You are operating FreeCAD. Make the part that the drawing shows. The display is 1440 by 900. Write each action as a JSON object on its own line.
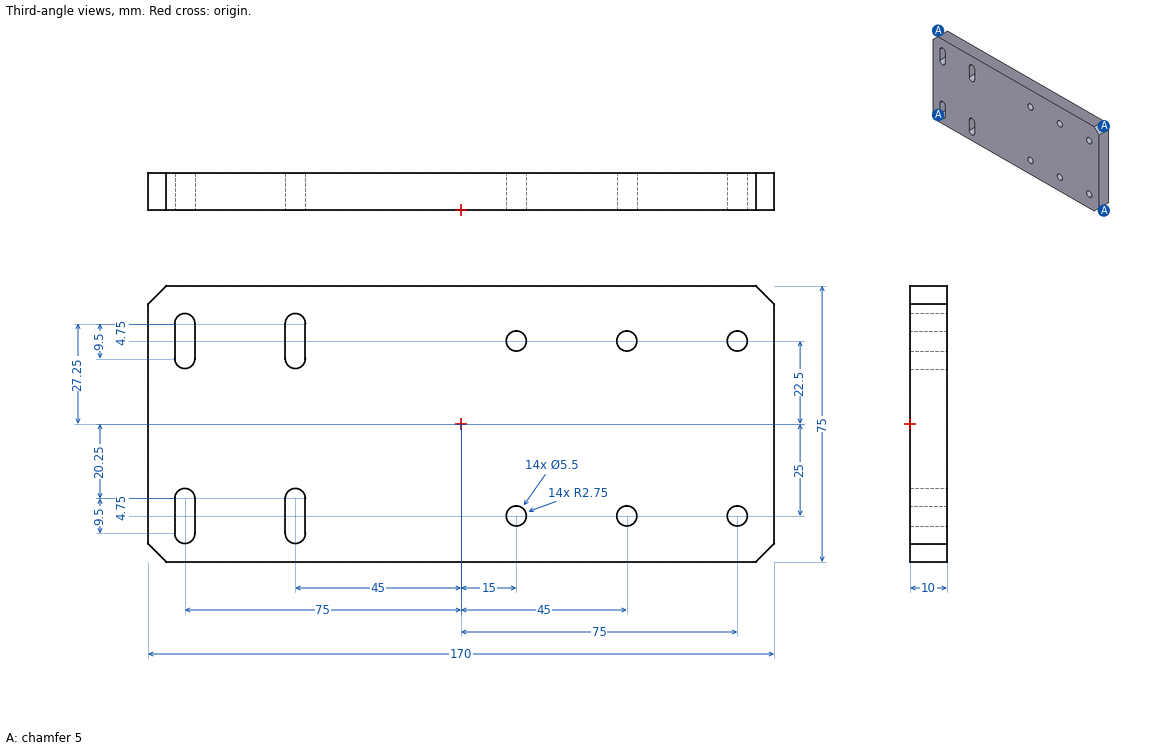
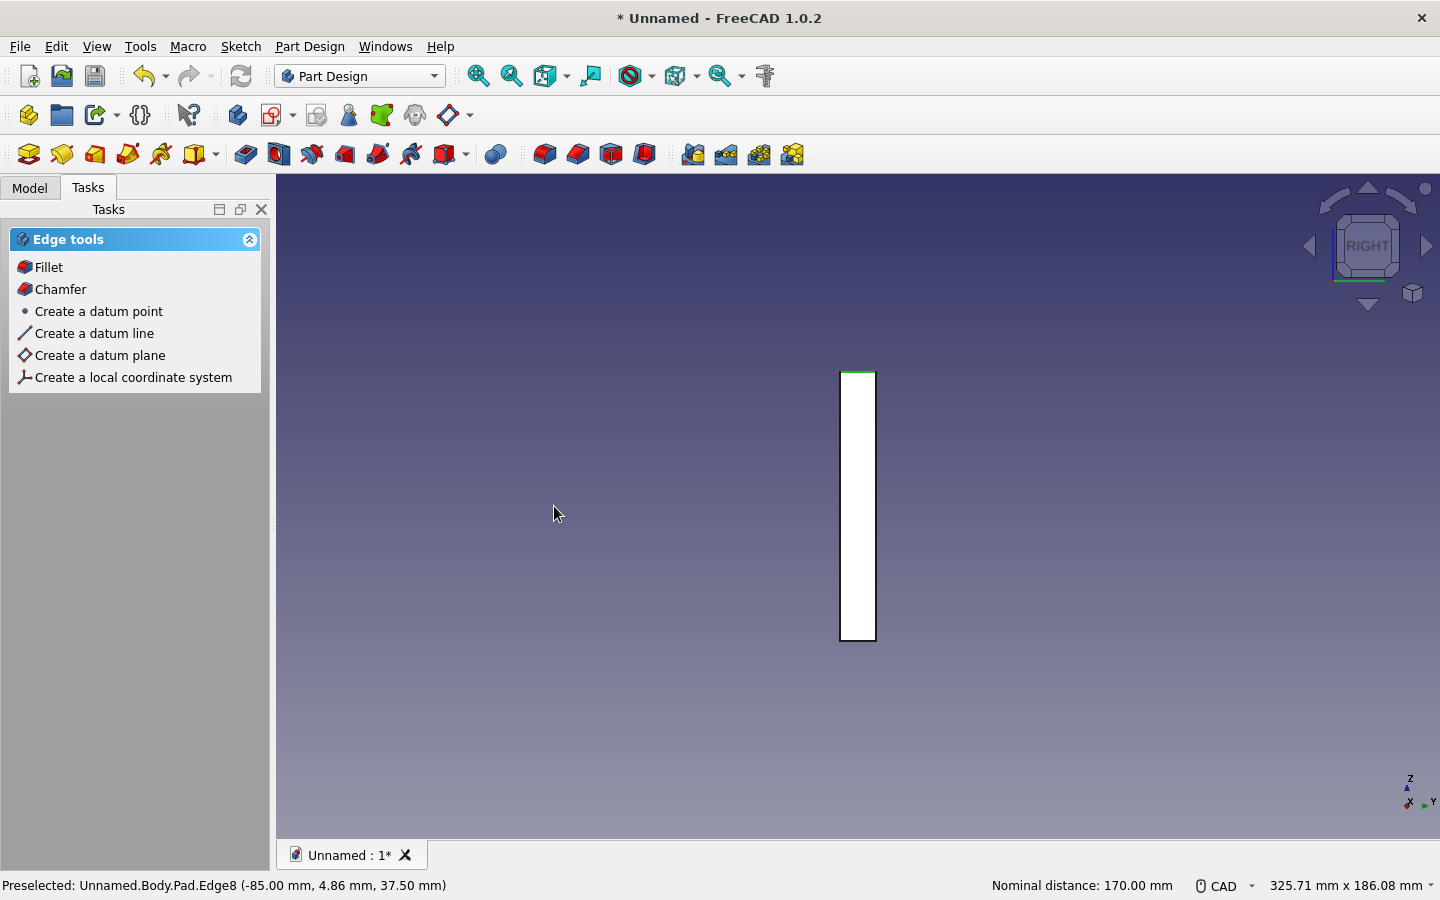
{"action": "key", "text": "v f"}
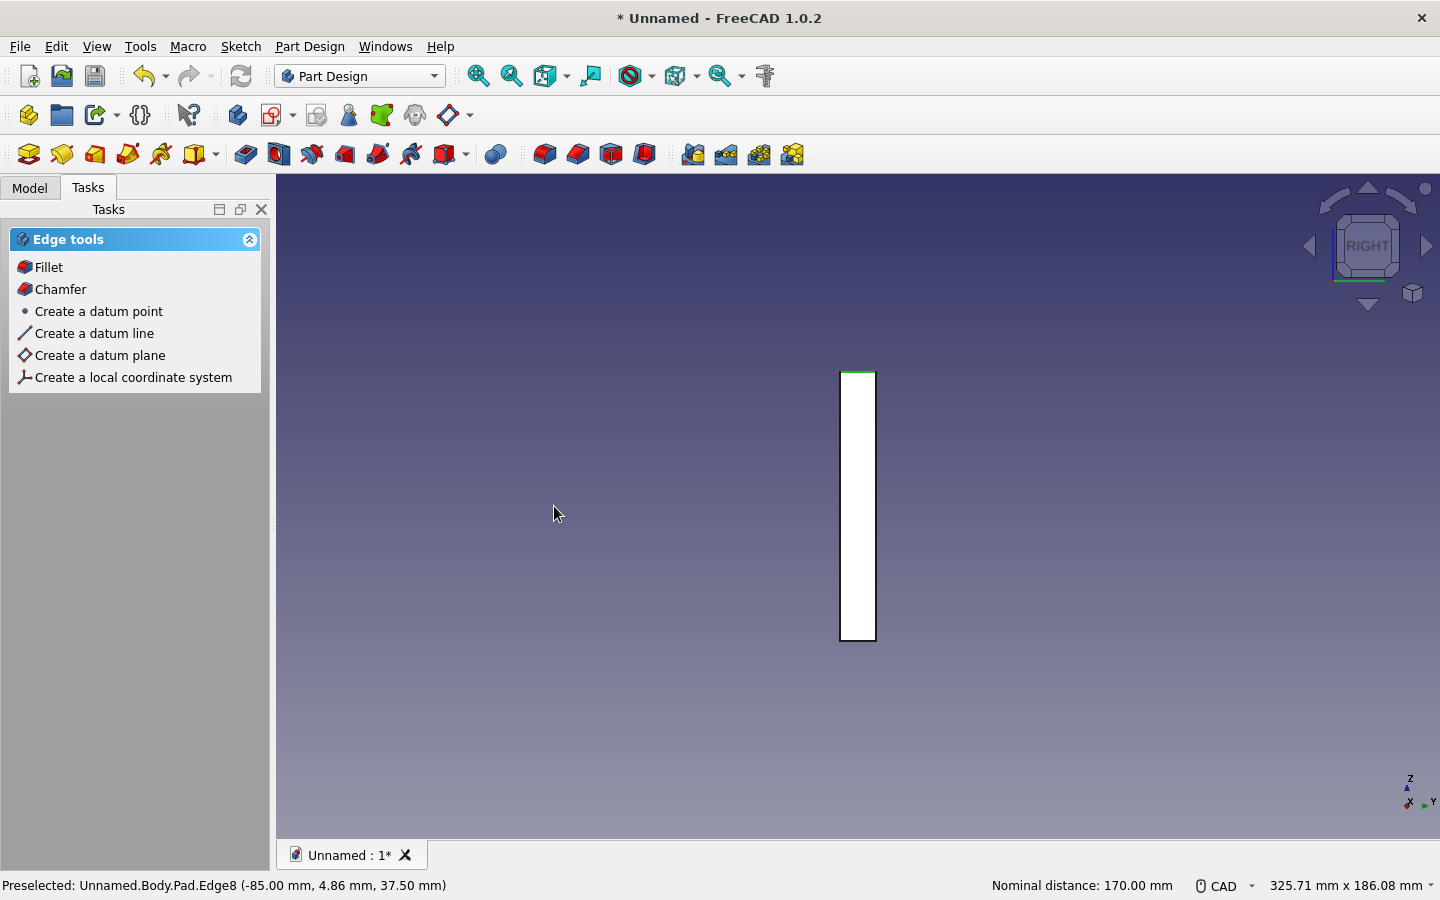
{"action": "left_click", "coordinate": [858, 640], "text": "ctrl"}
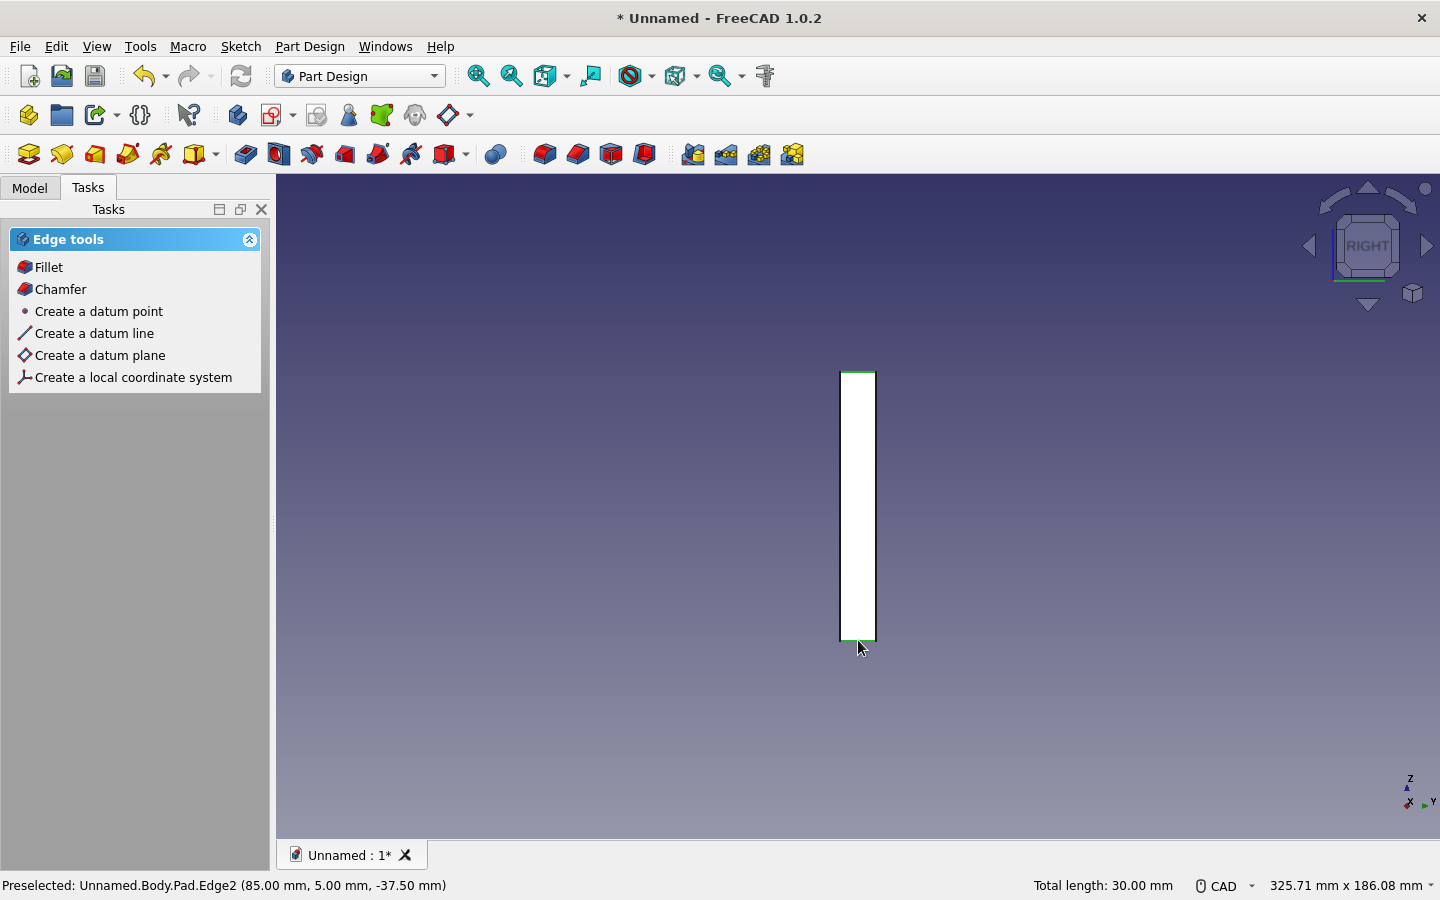
{"action": "key", "text": "5"}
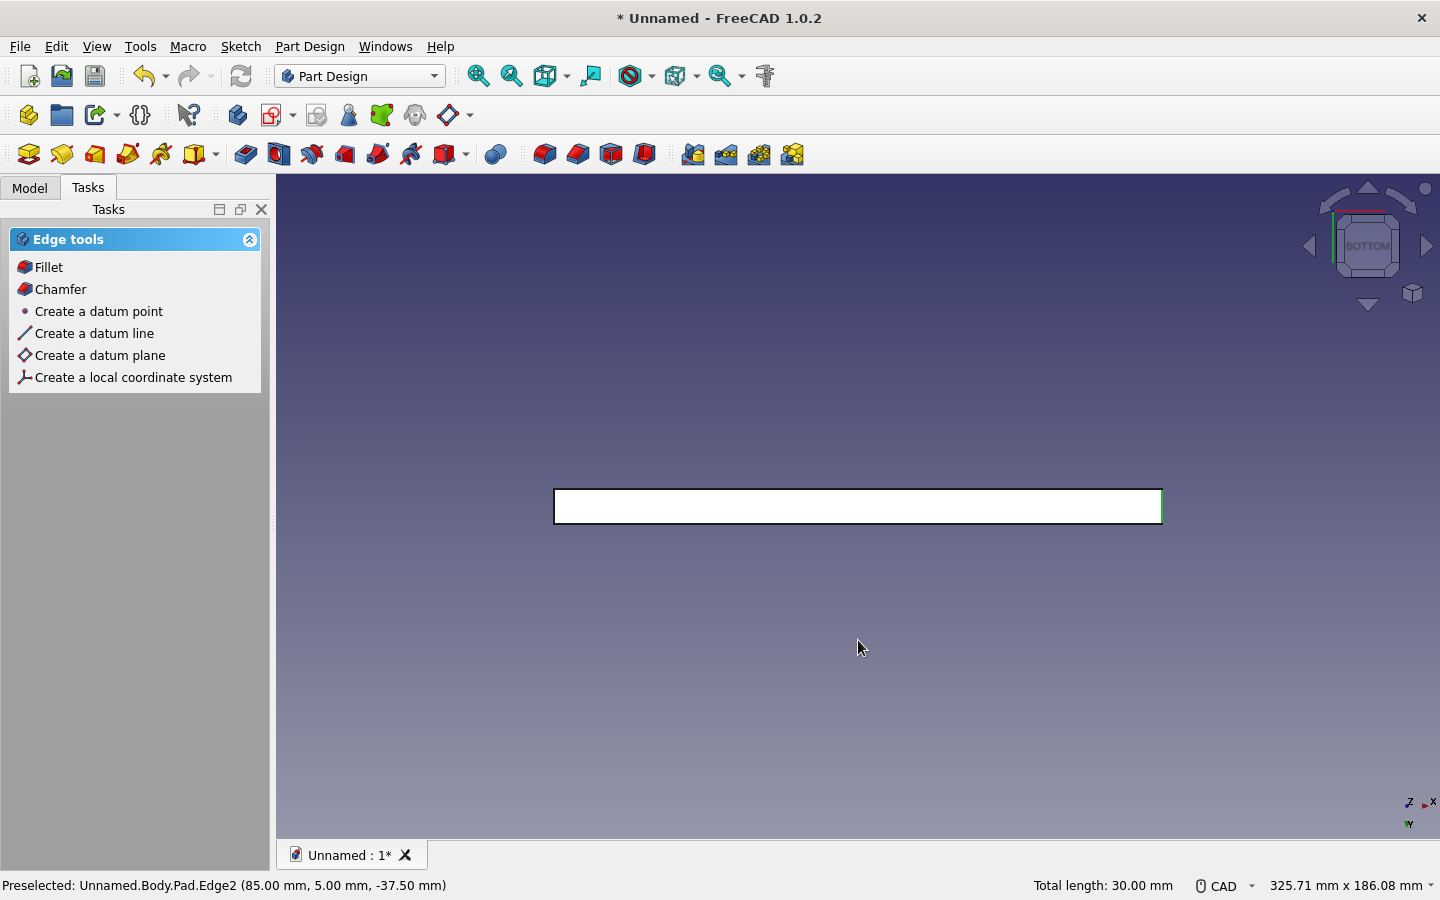
{"action": "left_click", "coordinate": [554, 505], "text": "ctrl"}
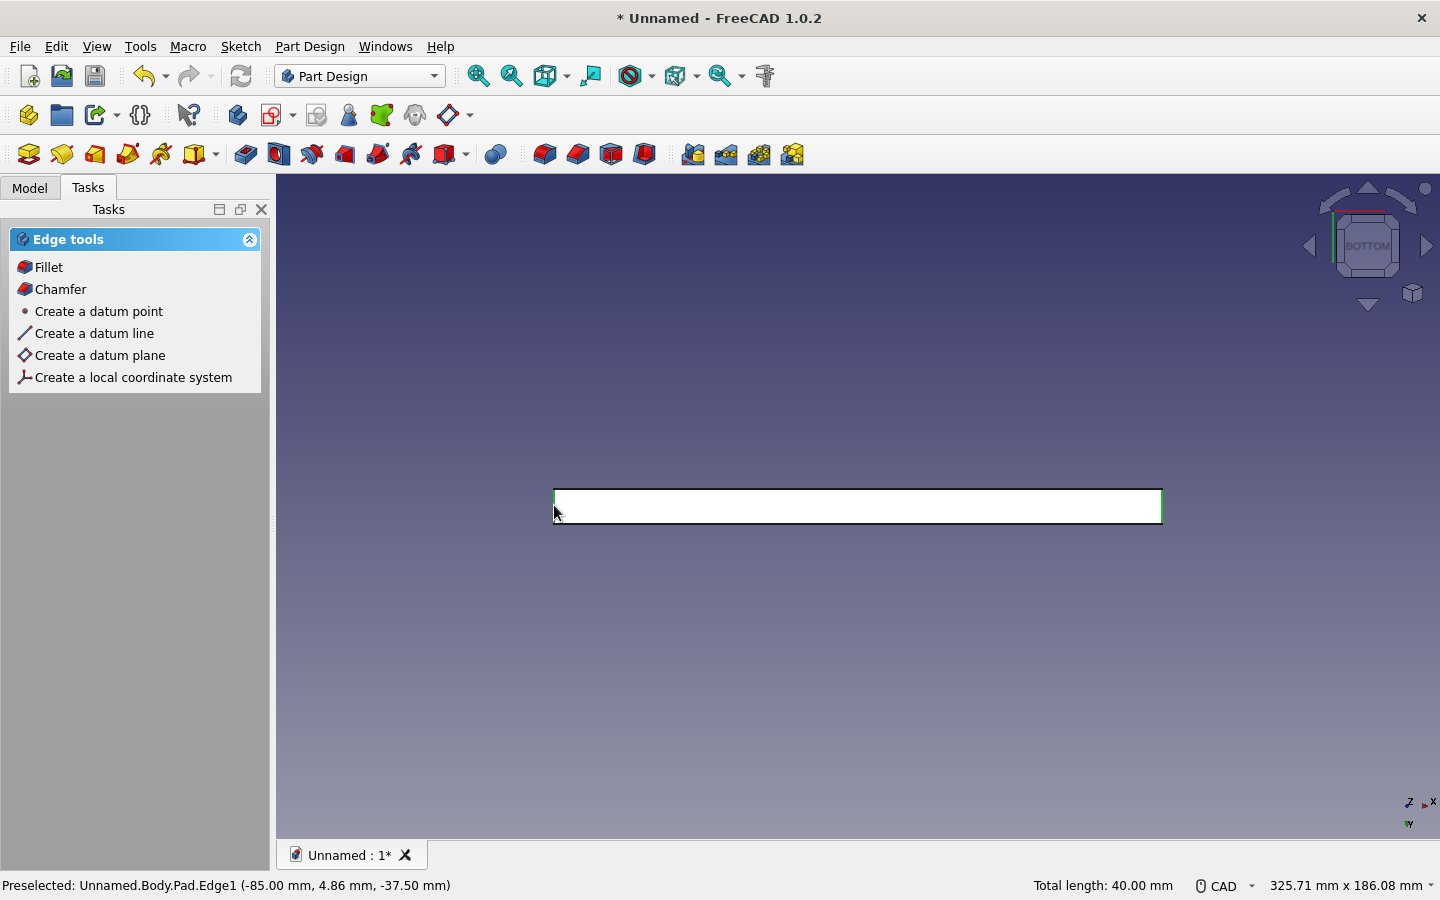
{"action": "left_click", "coordinate": [578, 154]}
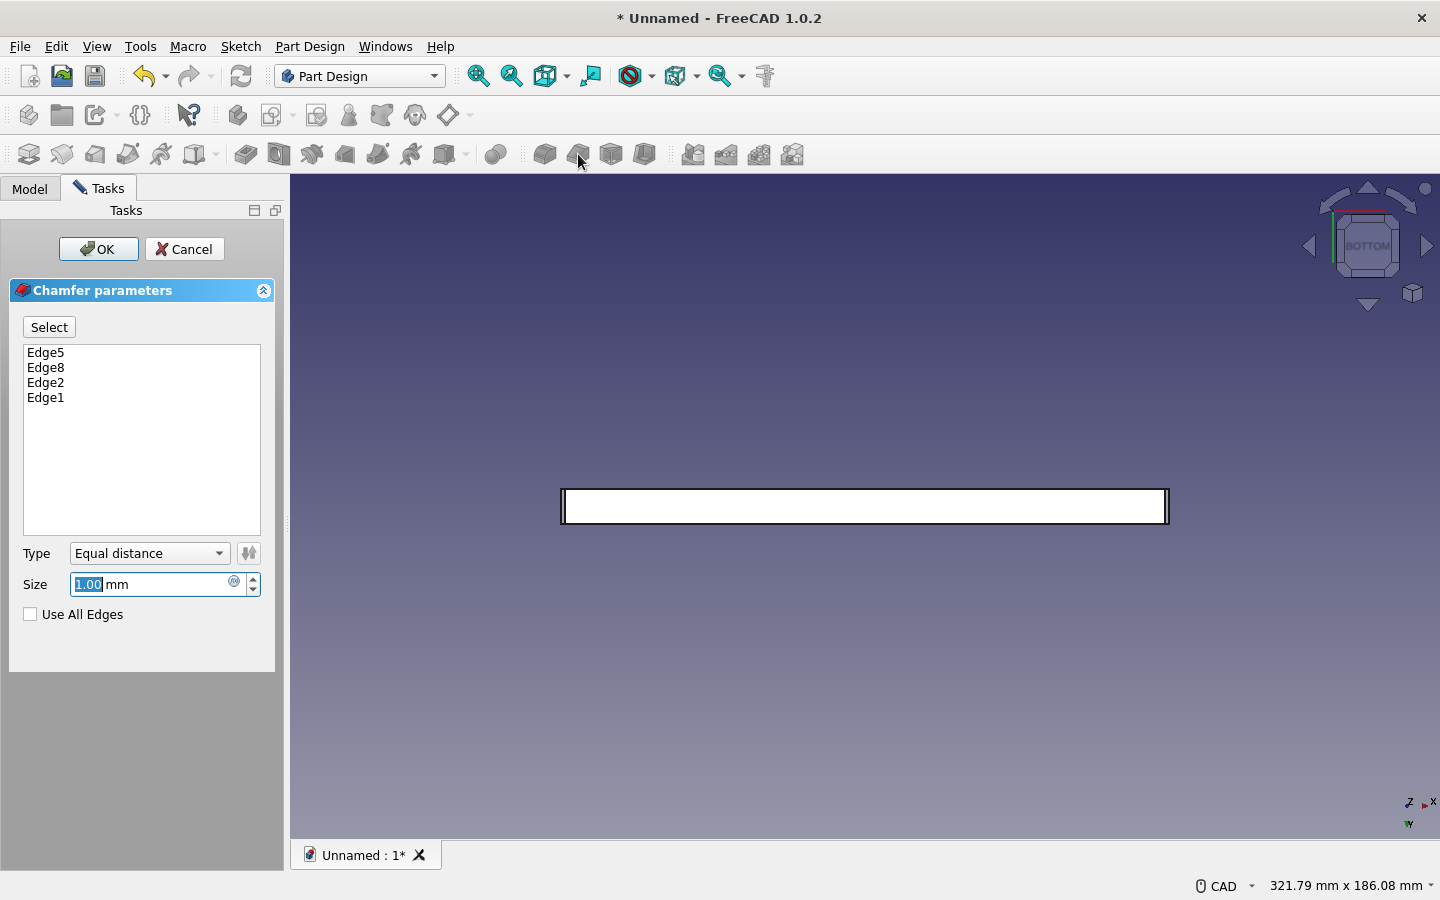
{"action": "type", "text": "5"}
{"action": "key", "text": "Tab"}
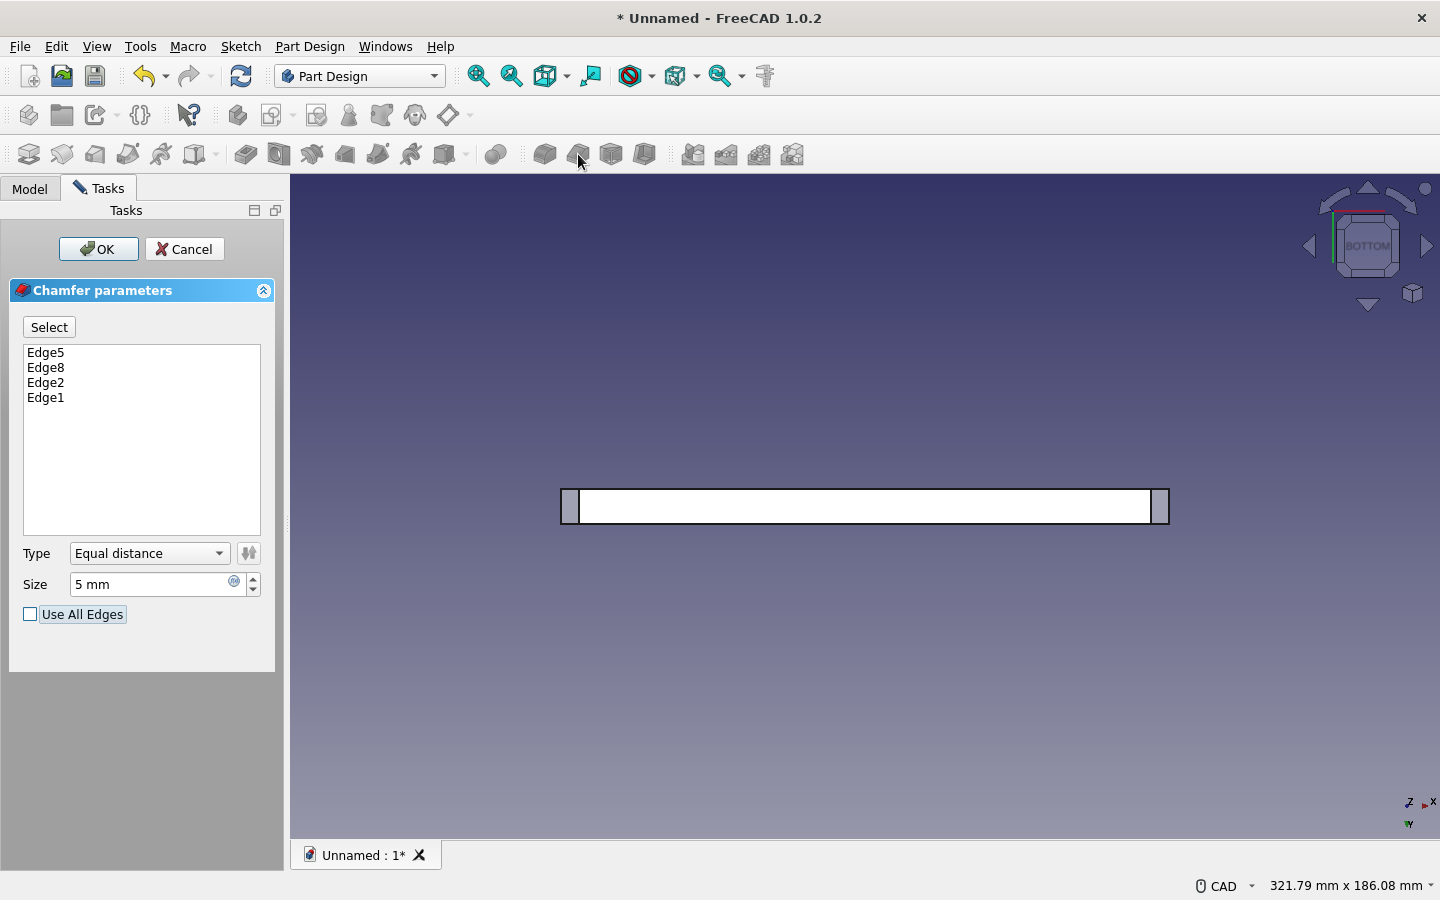
{"action": "left_click", "coordinate": [99, 249]}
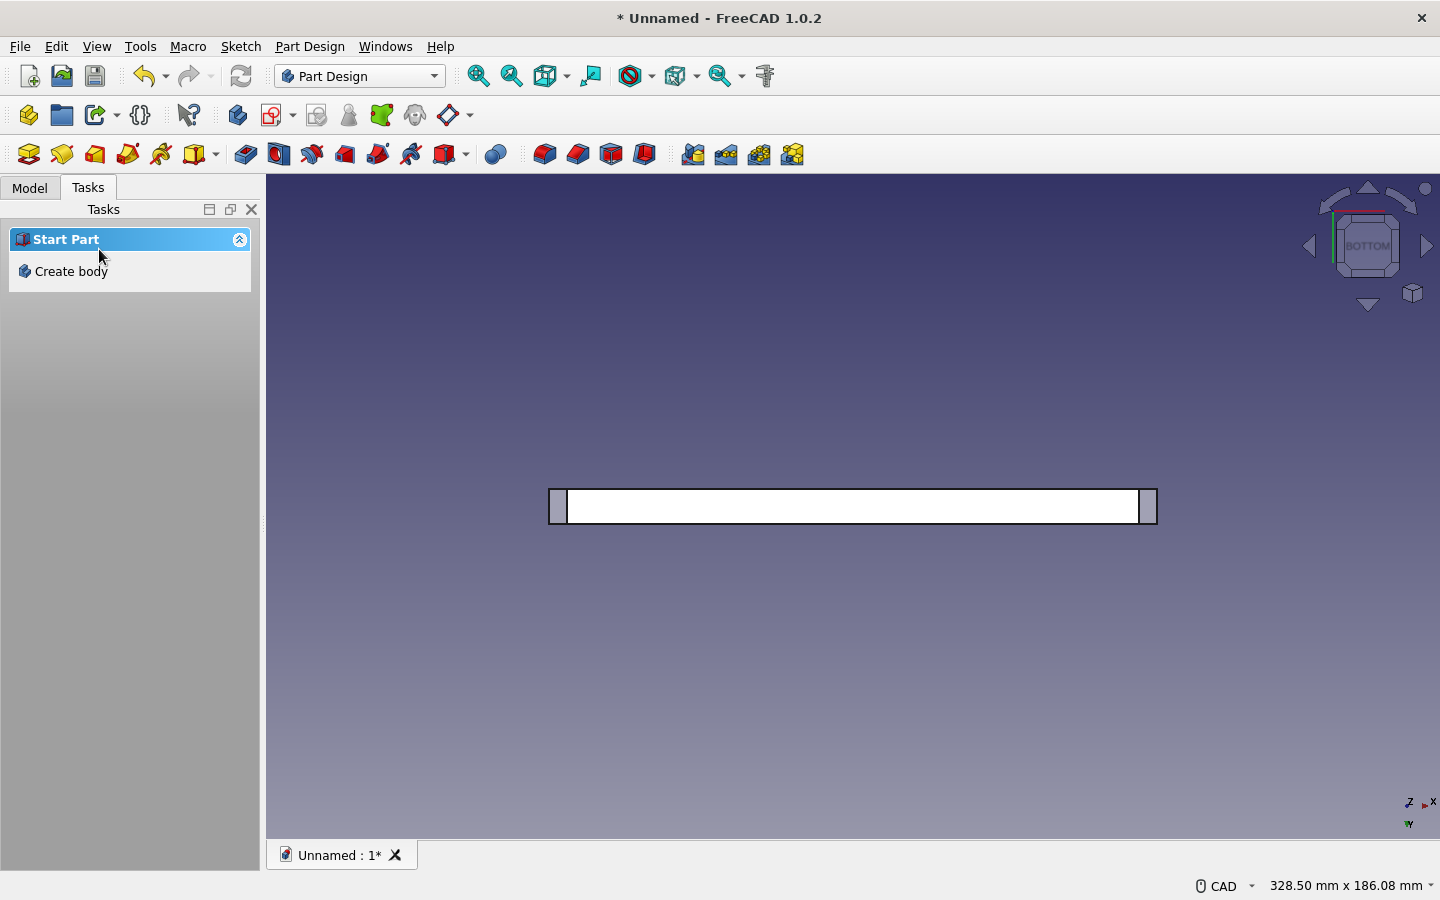
{"action": "key", "text": "4"}